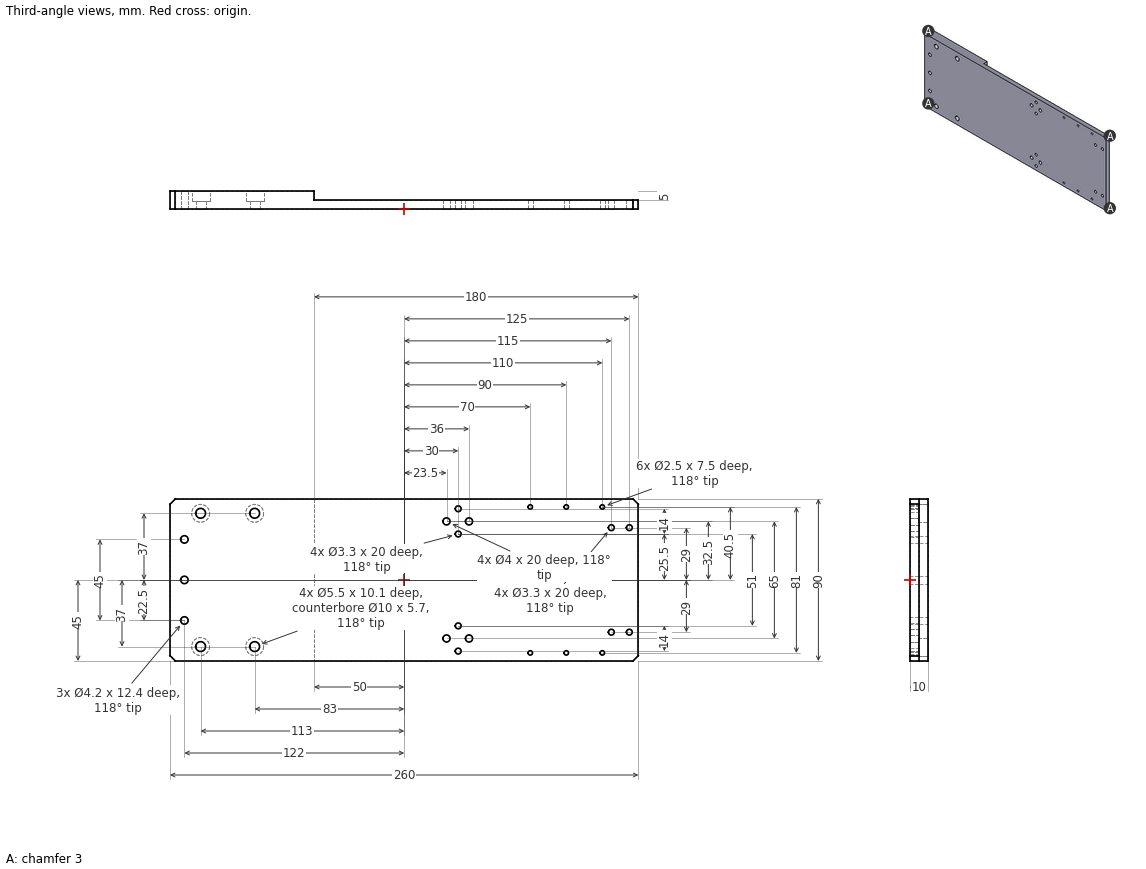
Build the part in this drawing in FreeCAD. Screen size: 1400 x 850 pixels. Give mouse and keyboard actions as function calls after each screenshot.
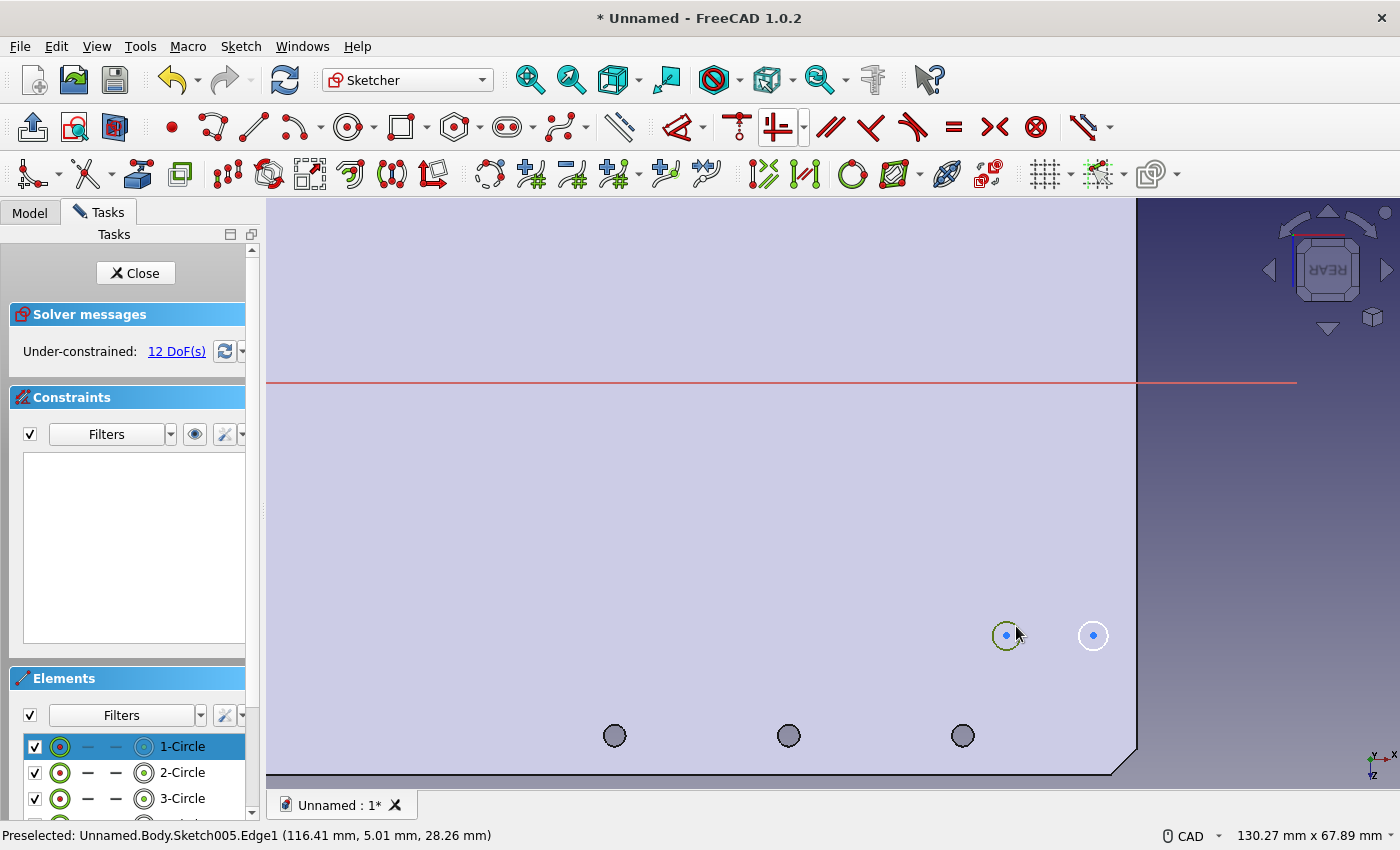
click(1103, 626)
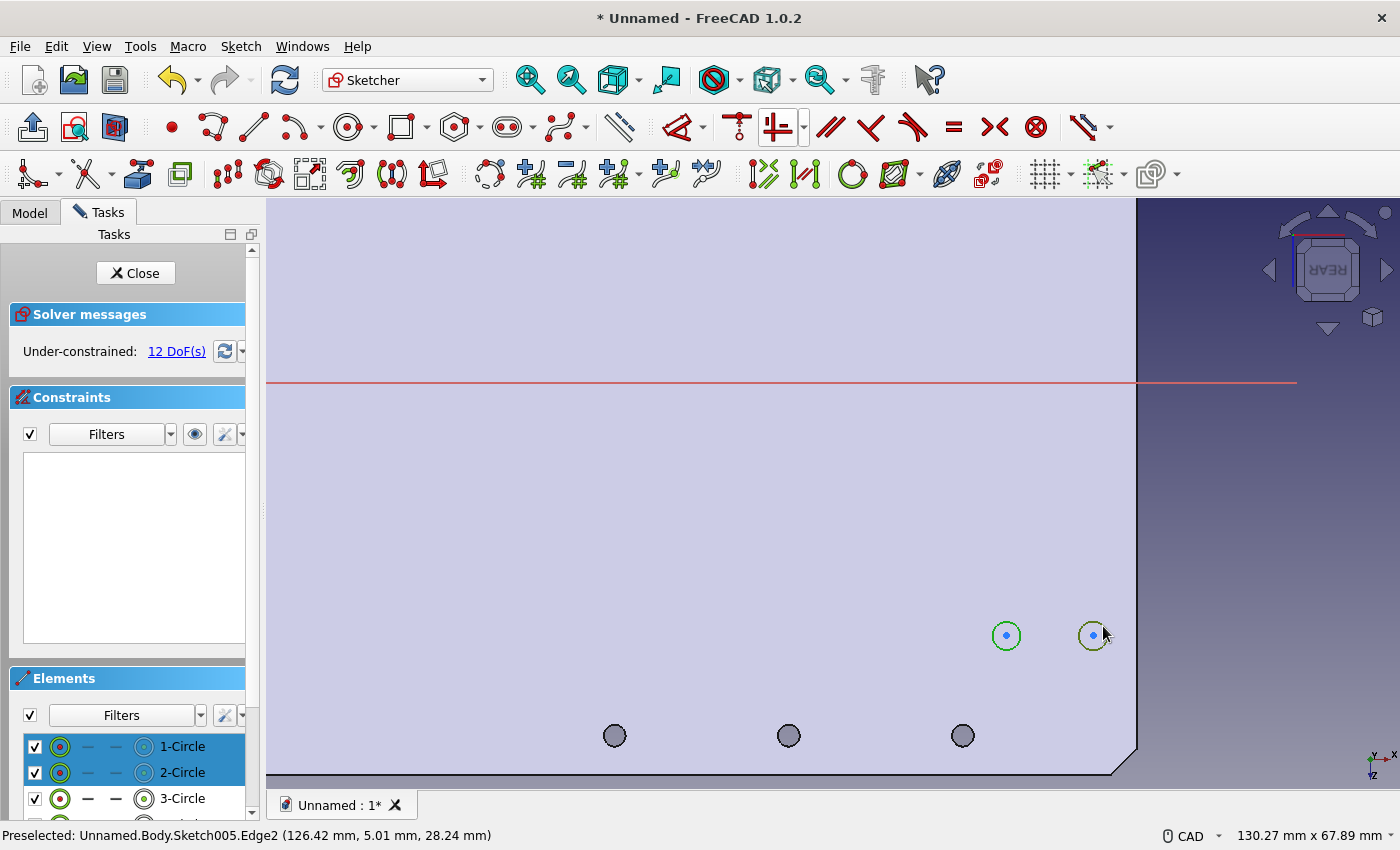
scroll(1017, 628, down, 3)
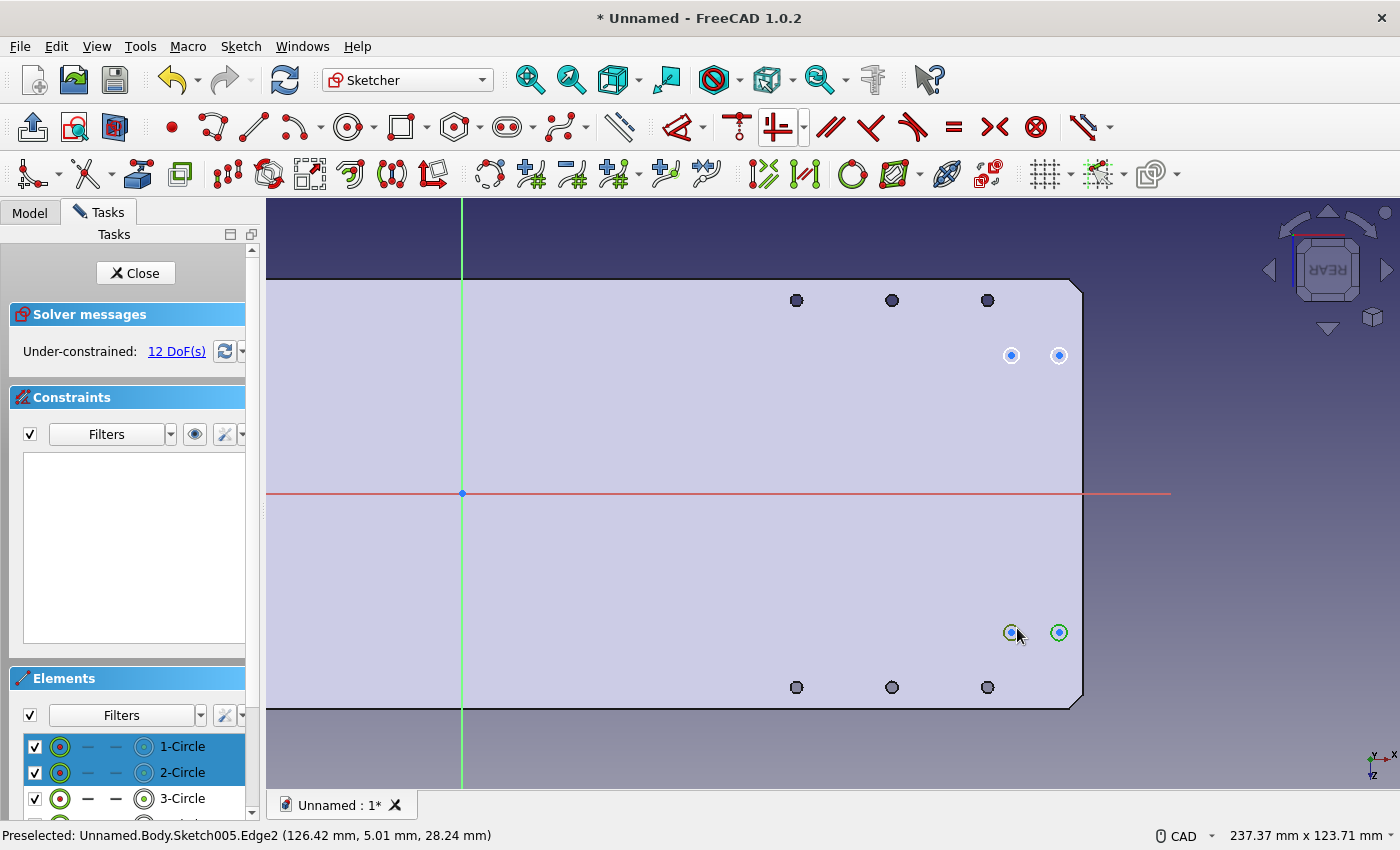
scroll(1017, 350, up, 3)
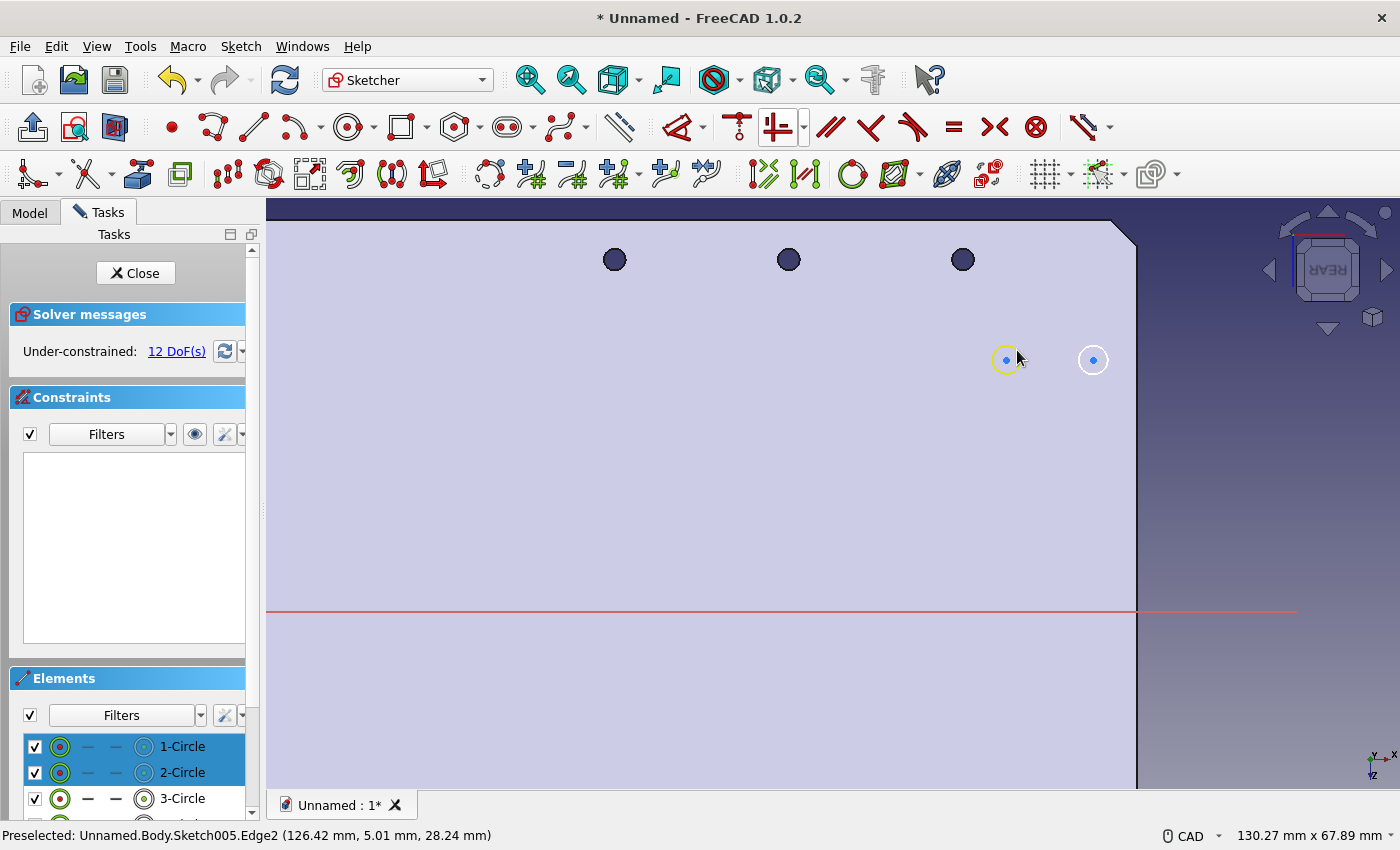
click(1016, 350)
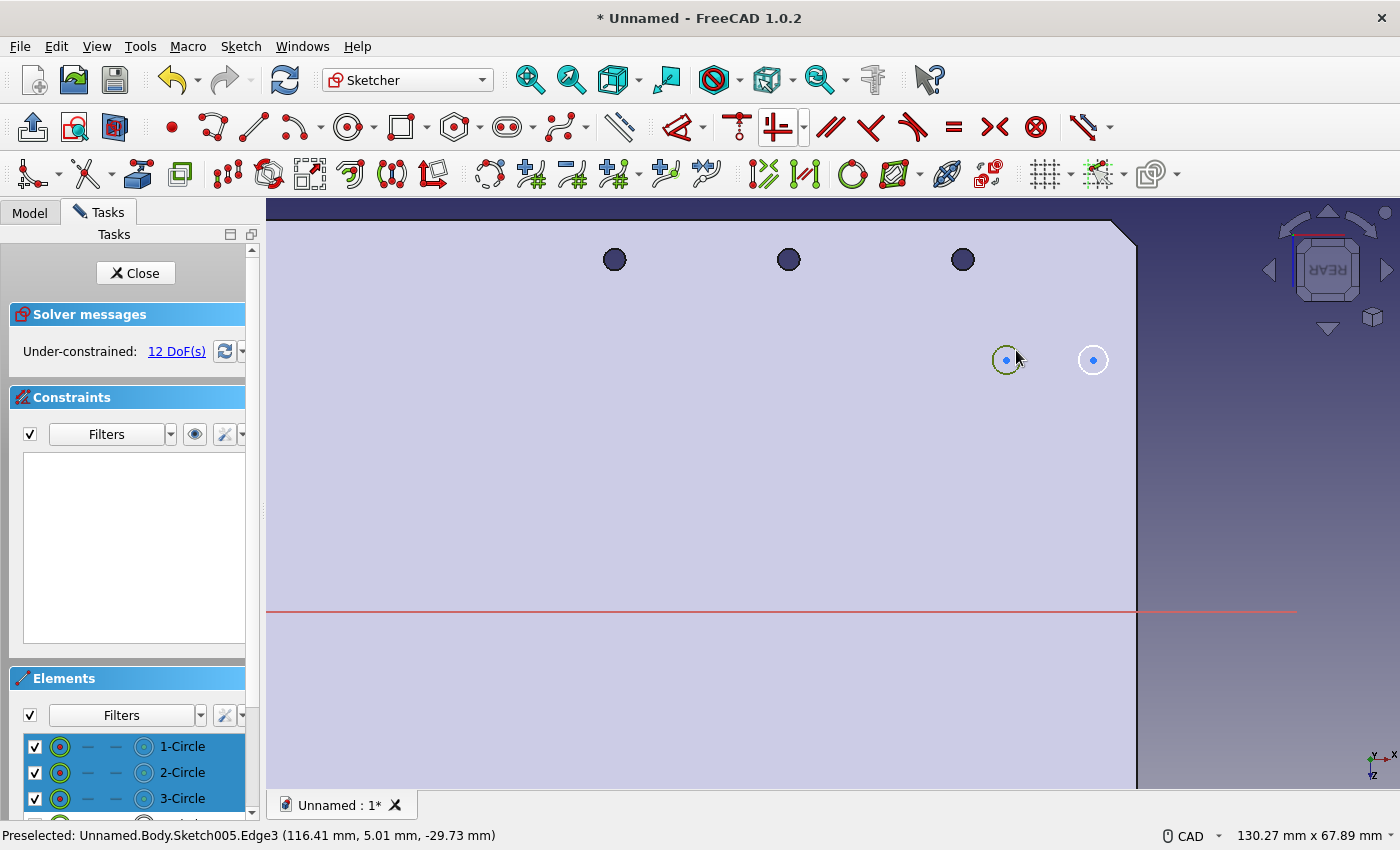
click(1103, 350)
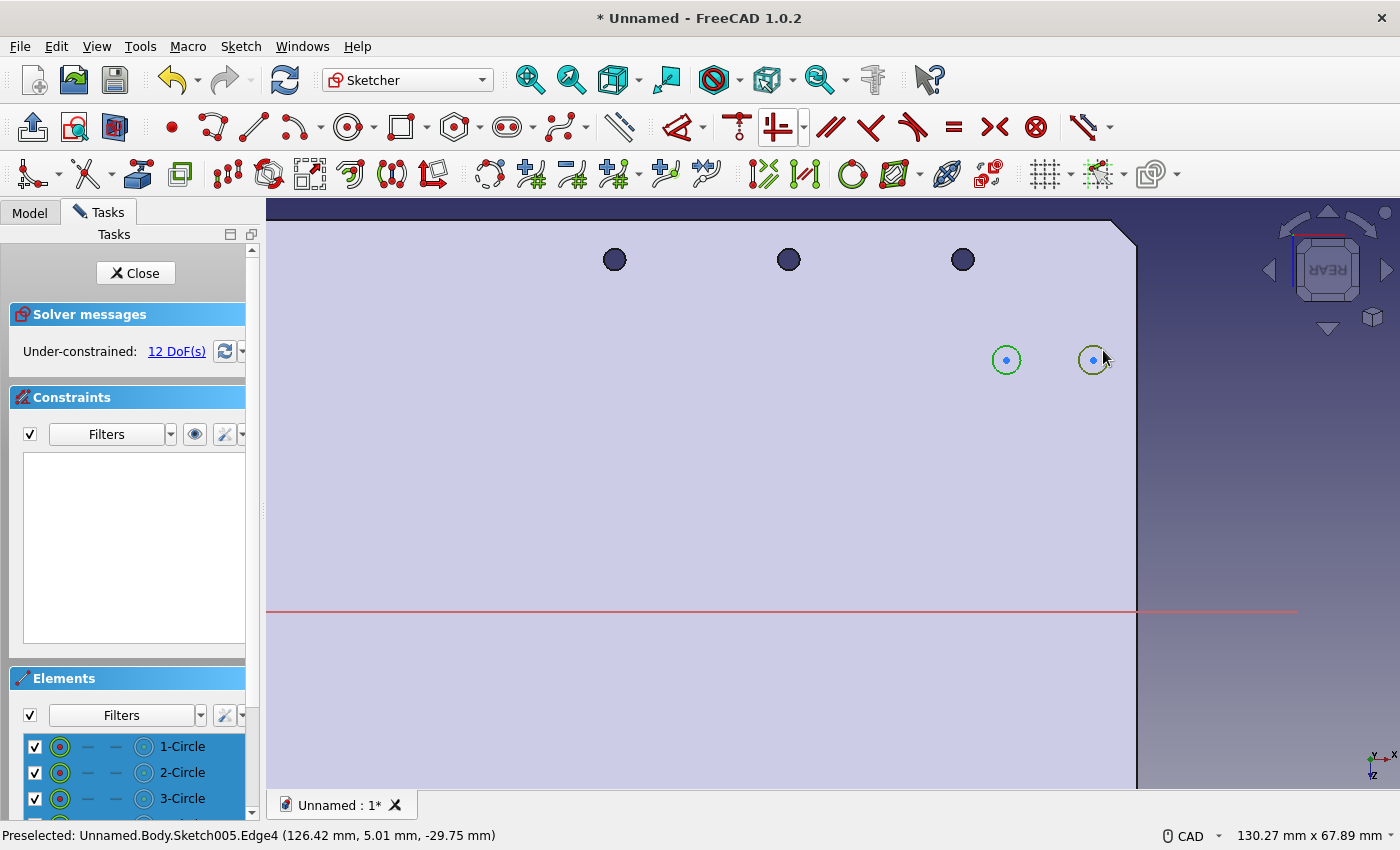
click(954, 128)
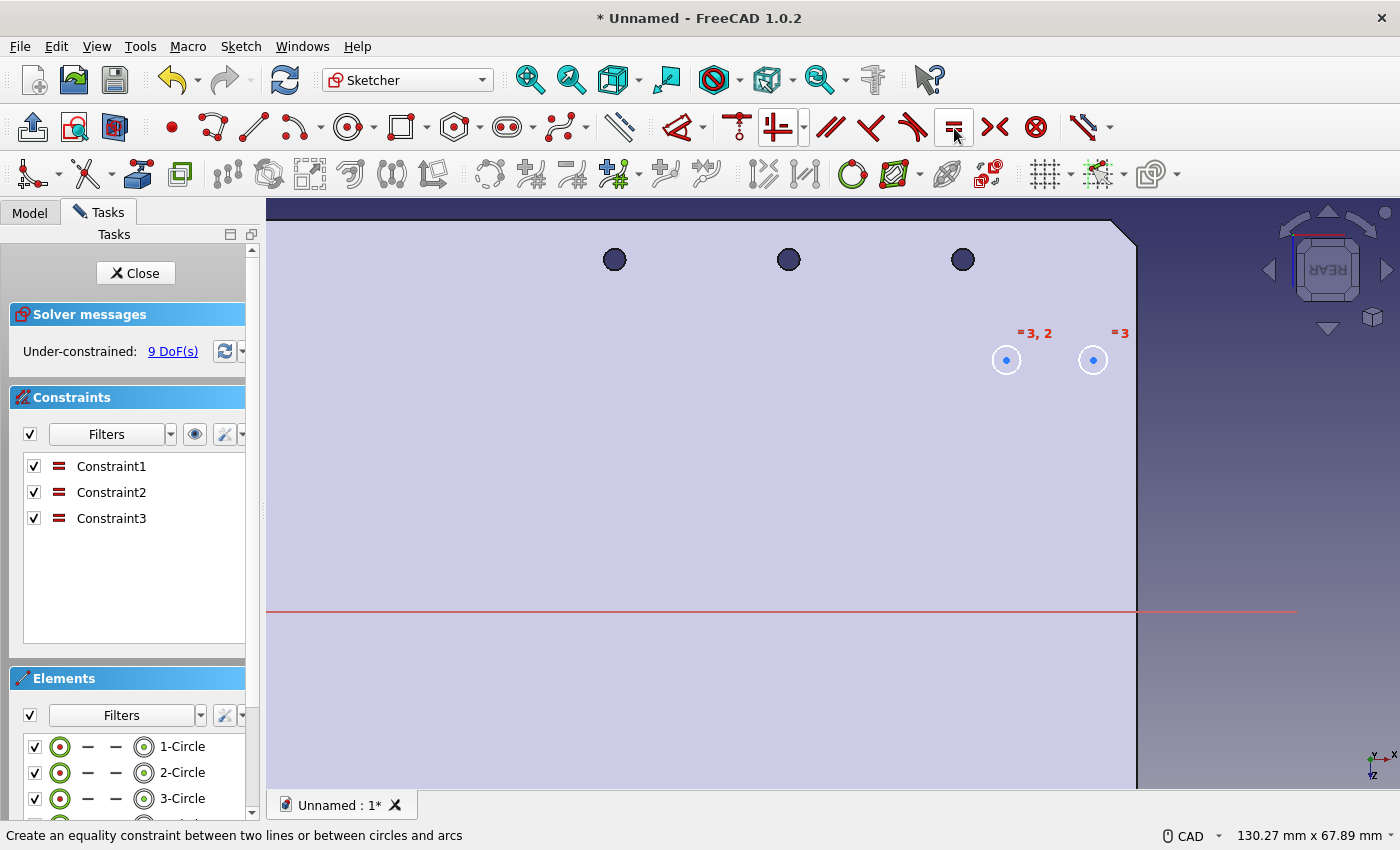
scroll(1017, 349, down, 3)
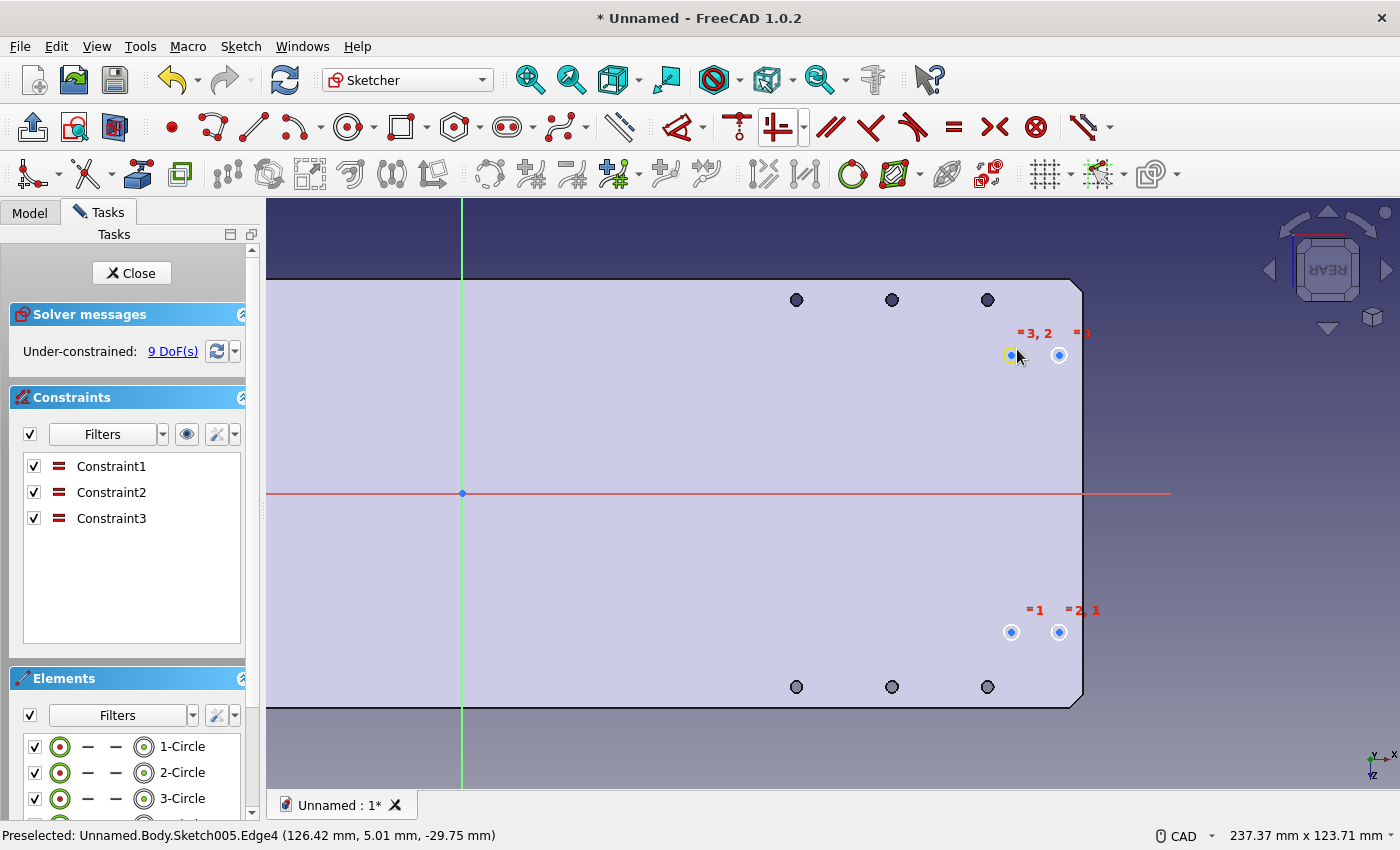
click(1012, 632)